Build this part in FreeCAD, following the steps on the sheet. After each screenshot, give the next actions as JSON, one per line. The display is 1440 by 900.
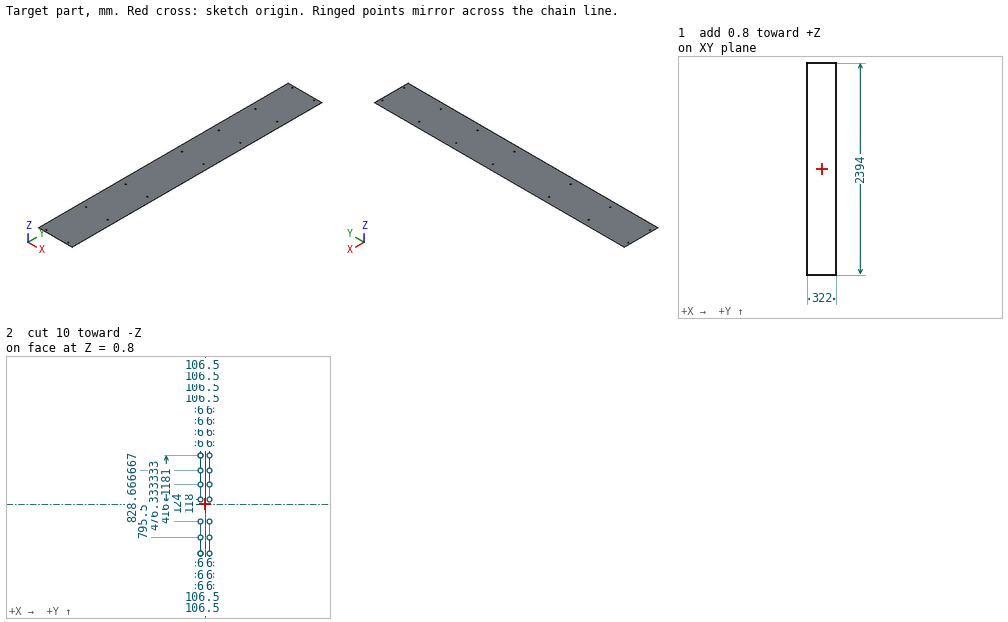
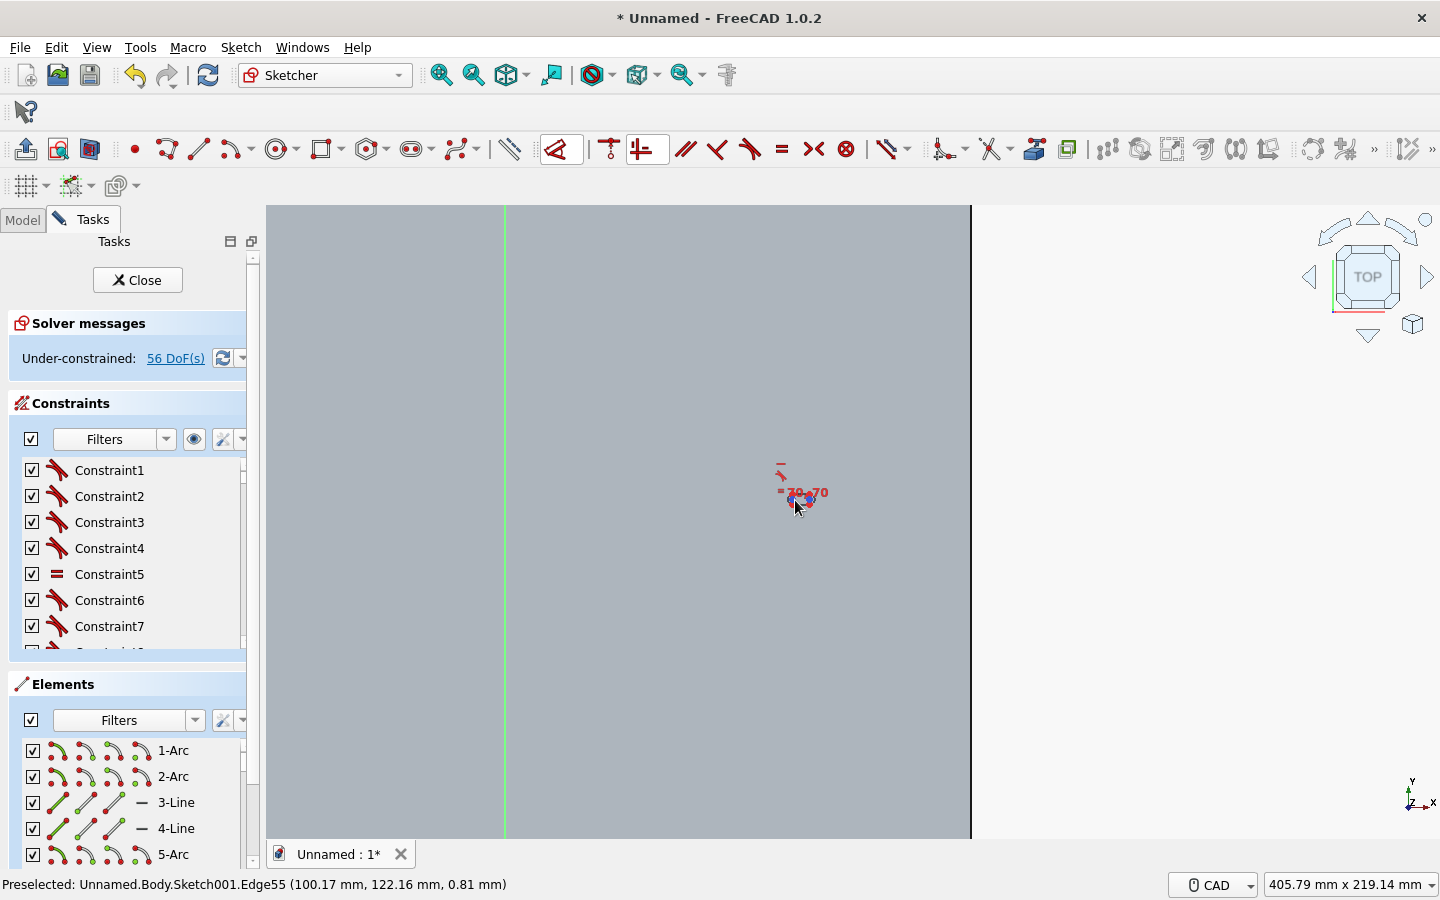
{"action": "scroll", "coordinate": [803, 501], "scroll_direction": "down", "scroll_amount": 14}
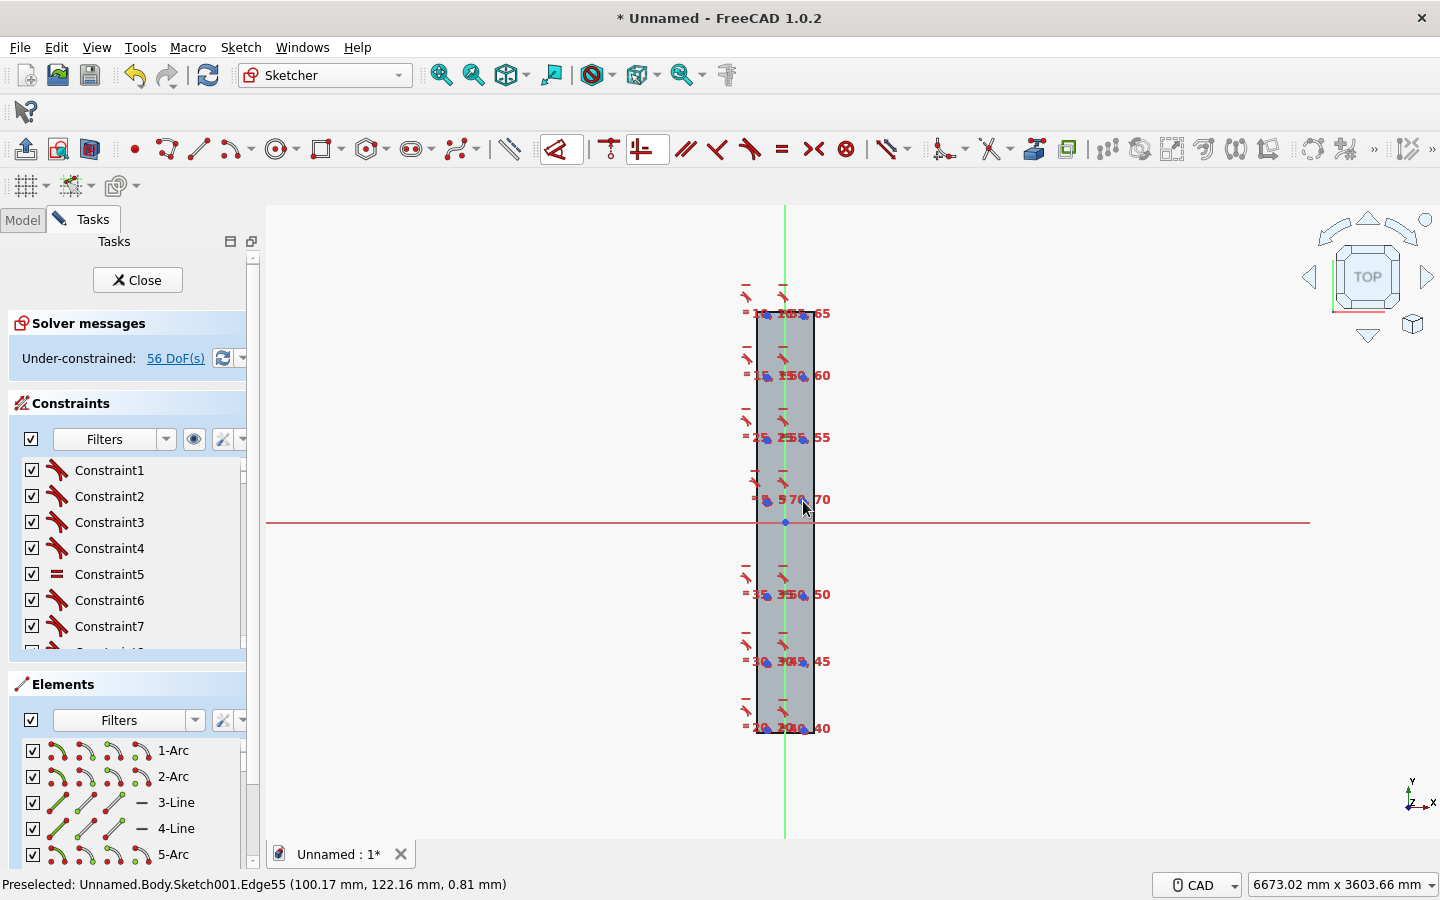
{"action": "scroll", "coordinate": [766, 501], "scroll_direction": "up", "scroll_amount": 13}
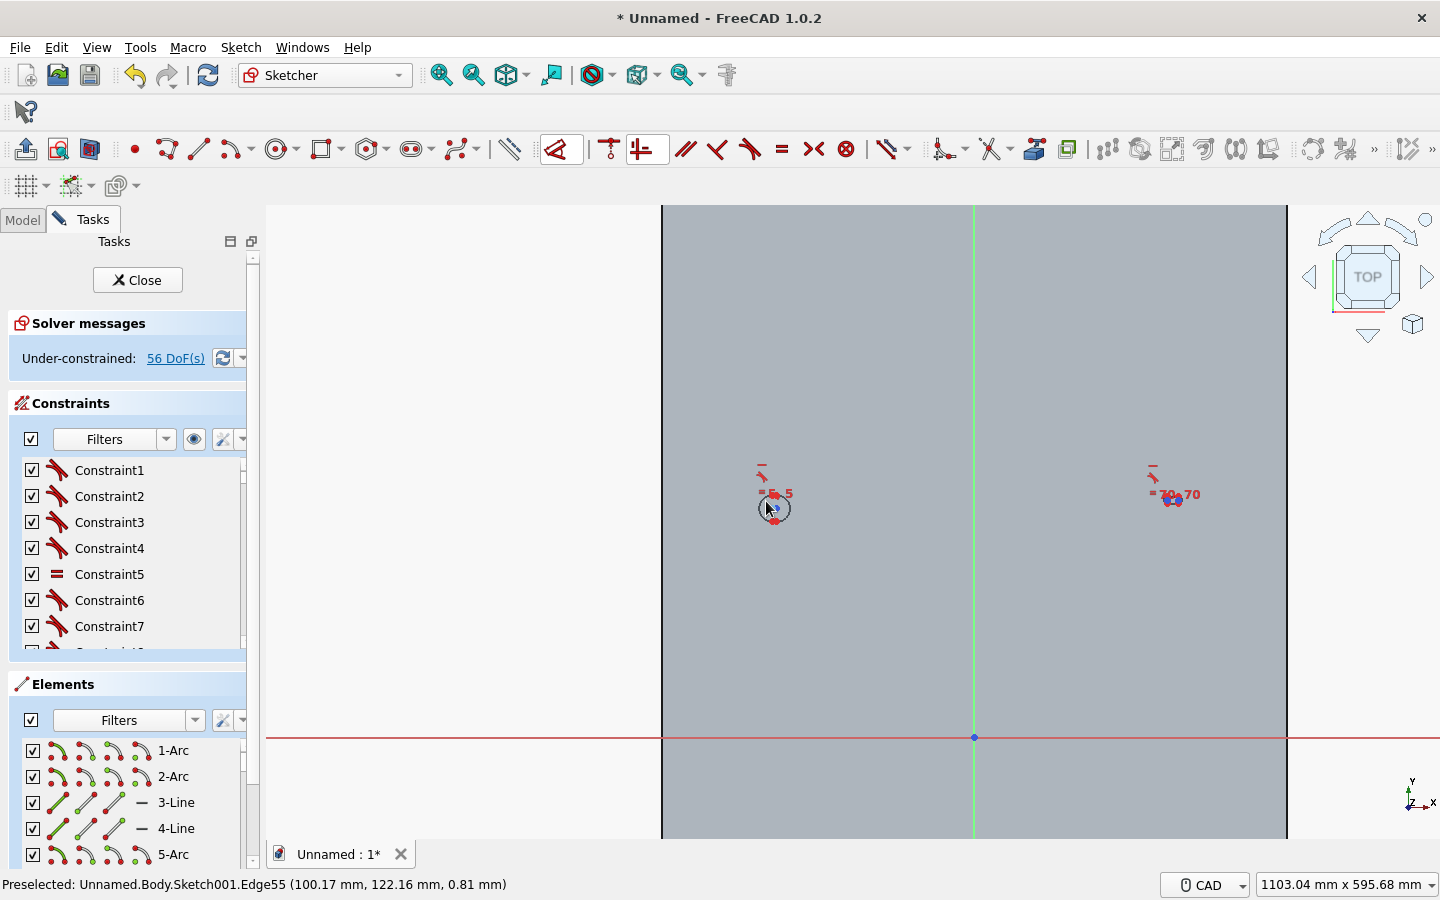
{"action": "left_click", "coordinate": [761, 501]}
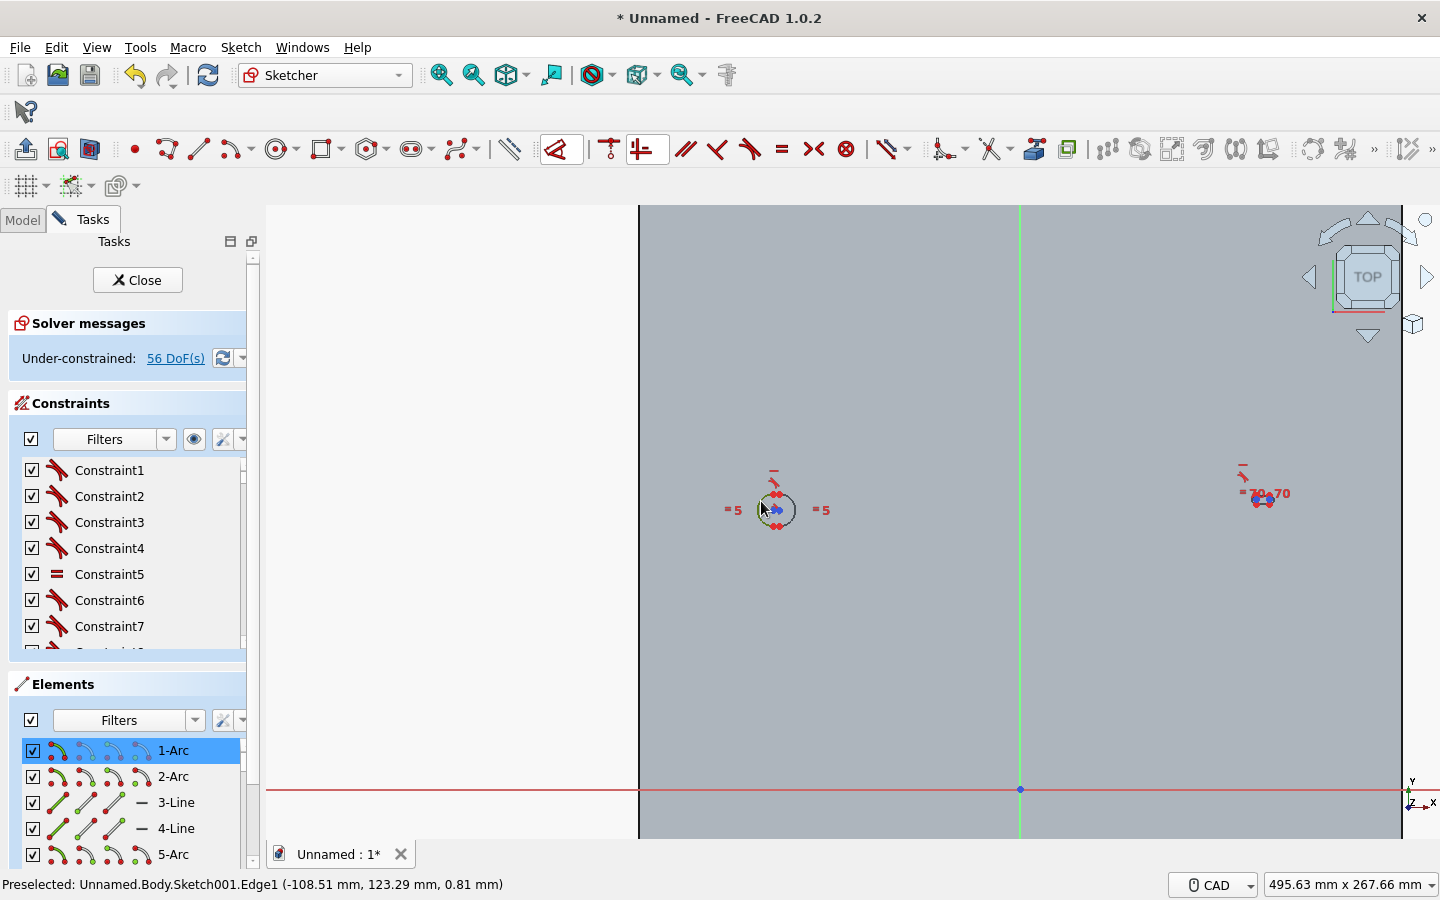
{"action": "scroll", "coordinate": [766, 501], "scroll_direction": "down", "scroll_amount": 13}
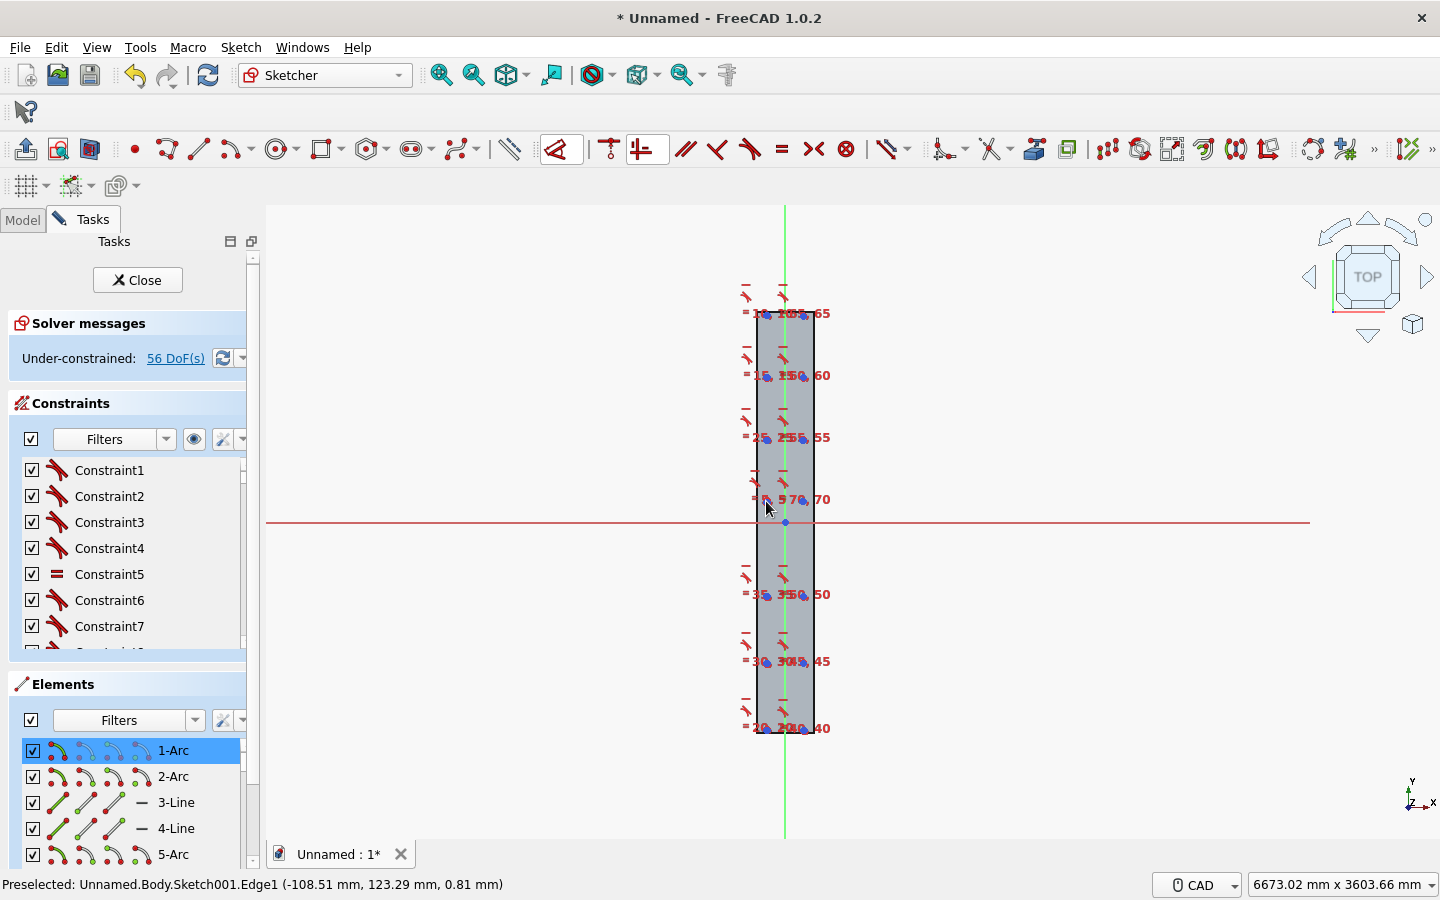
{"action": "scroll", "coordinate": [766, 315], "scroll_direction": "up", "scroll_amount": 14}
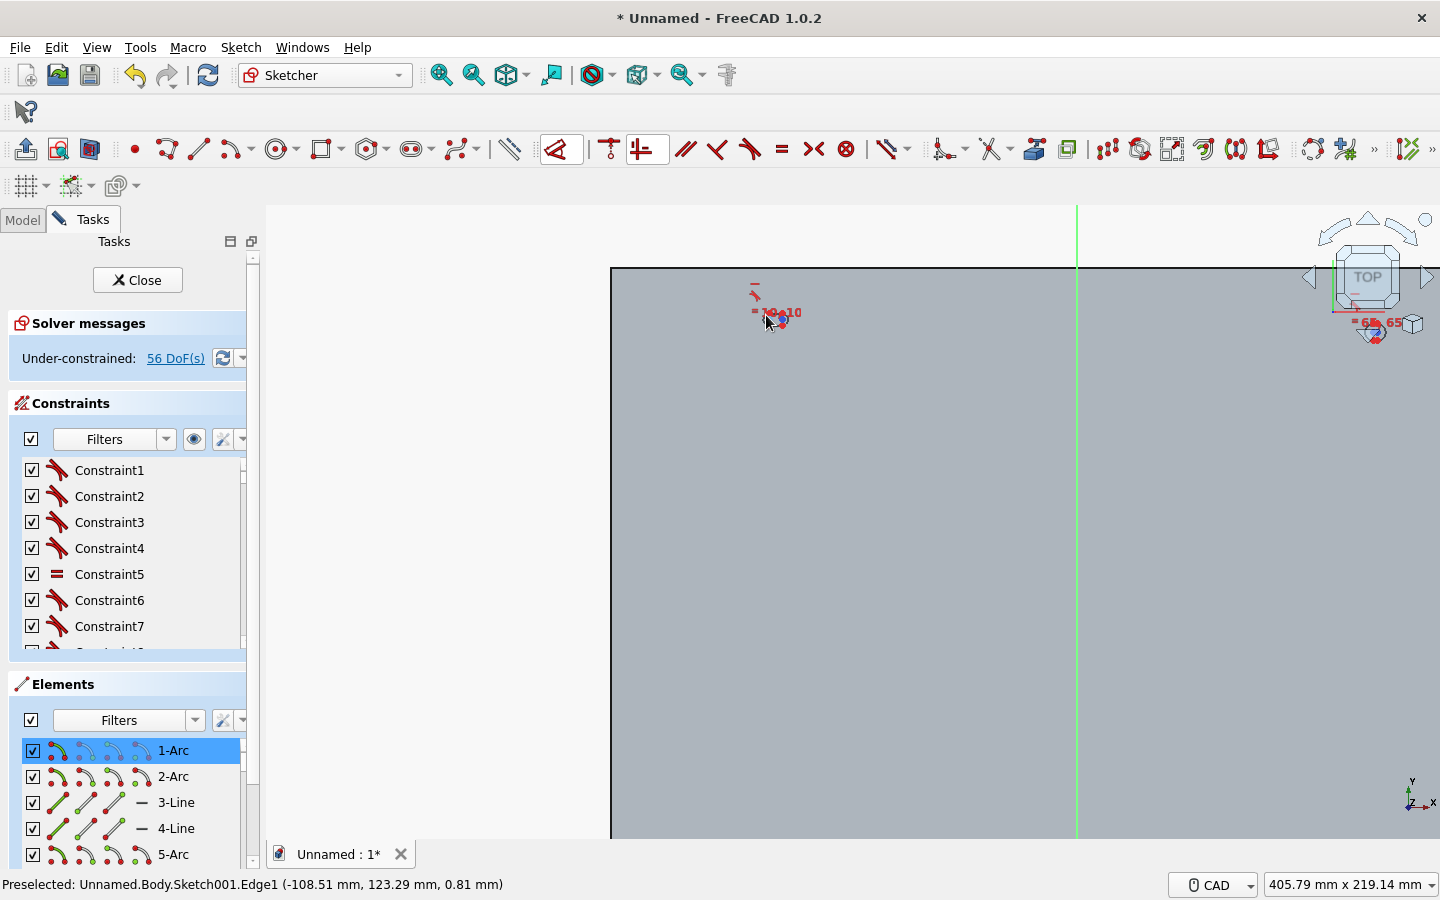
{"action": "left_click", "coordinate": [763, 320]}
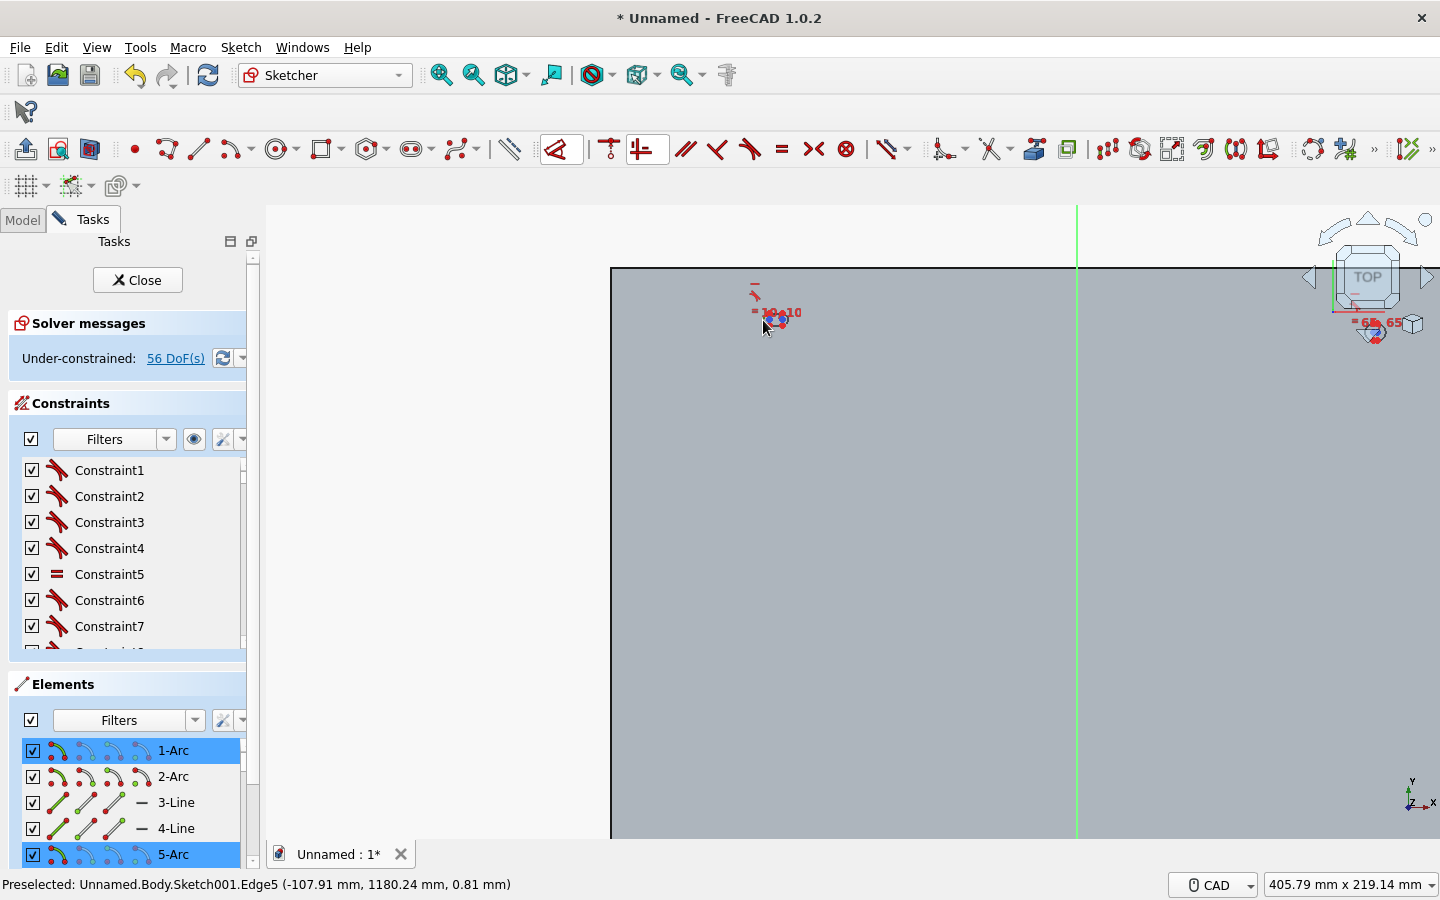
{"action": "scroll", "coordinate": [766, 314], "scroll_direction": "down", "scroll_amount": 14}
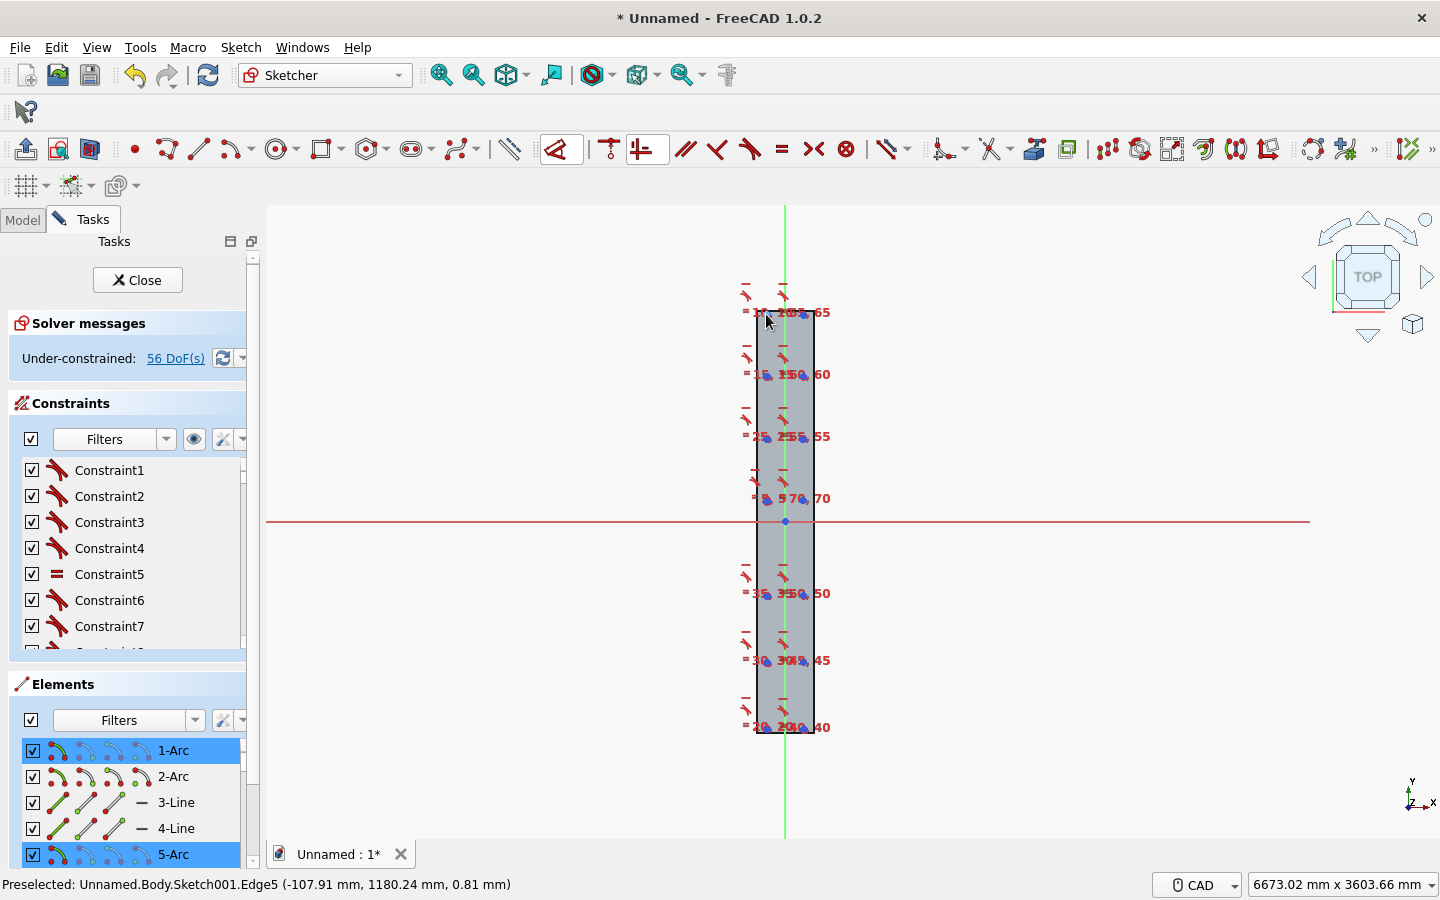
{"action": "scroll", "coordinate": [766, 377], "scroll_direction": "up", "scroll_amount": 14}